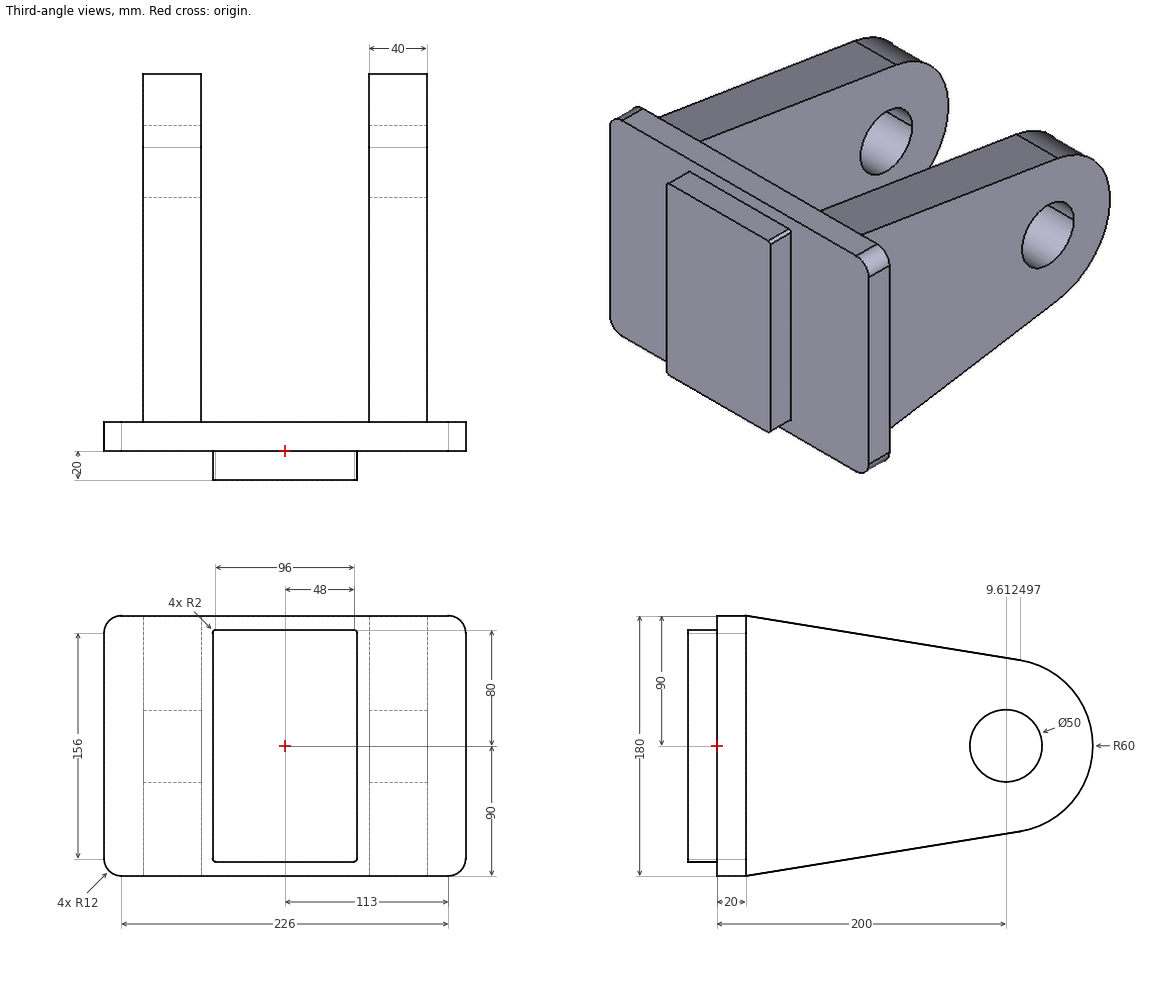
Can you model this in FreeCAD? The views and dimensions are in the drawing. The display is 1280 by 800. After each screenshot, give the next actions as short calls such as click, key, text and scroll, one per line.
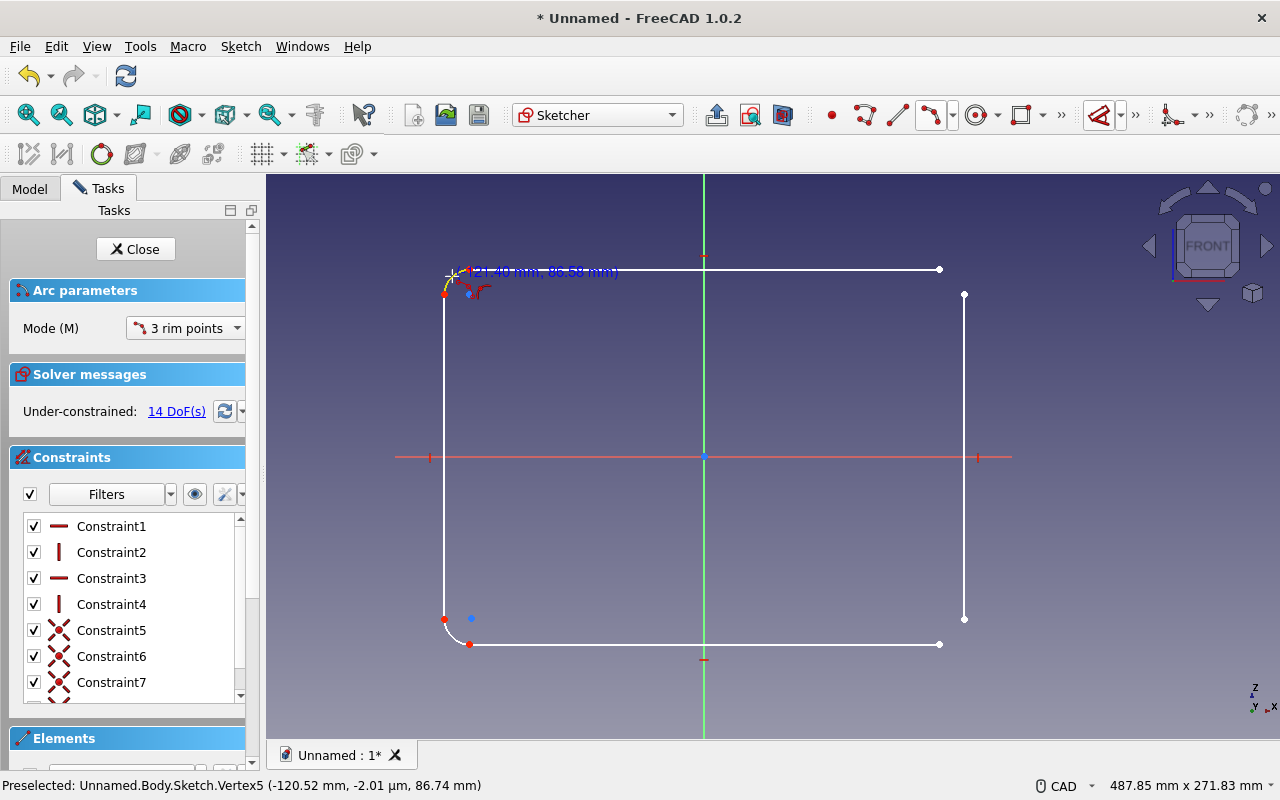
click(939, 270)
click(964, 295)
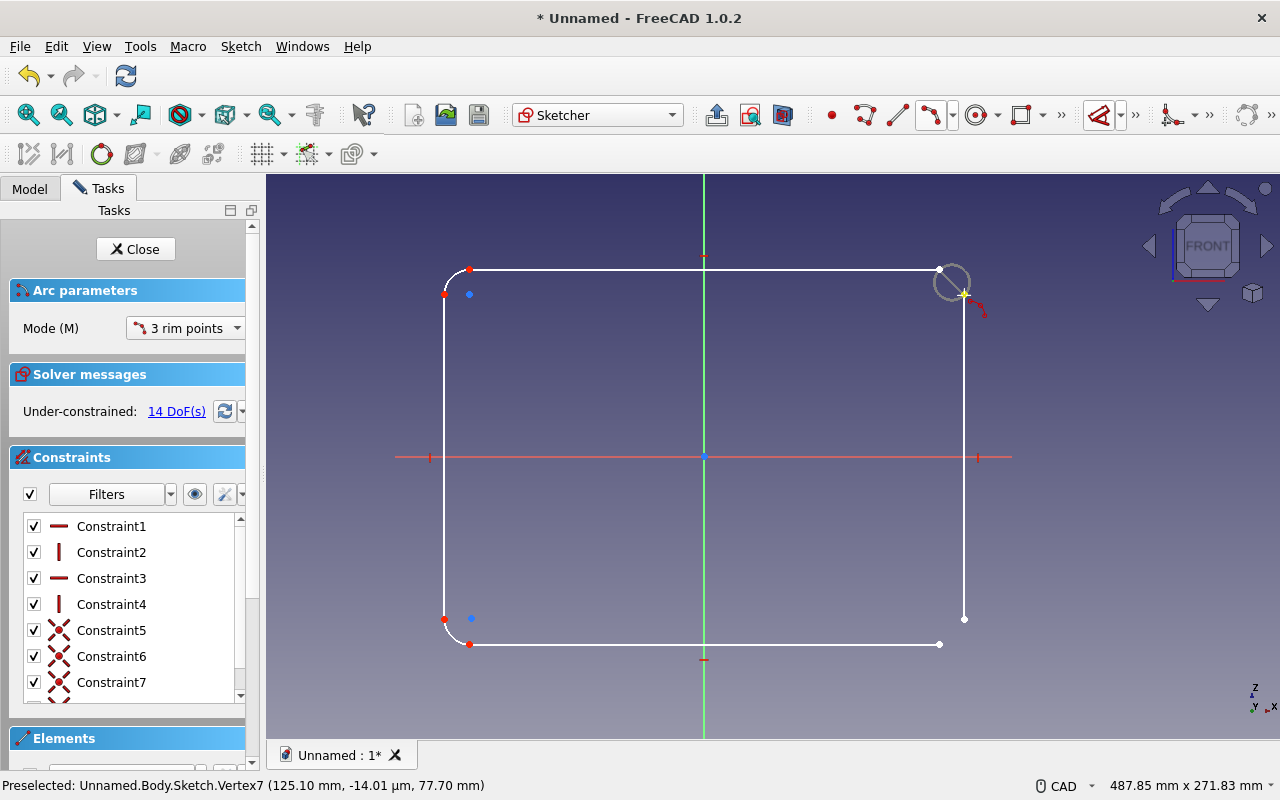
scroll(957, 277, up, 4)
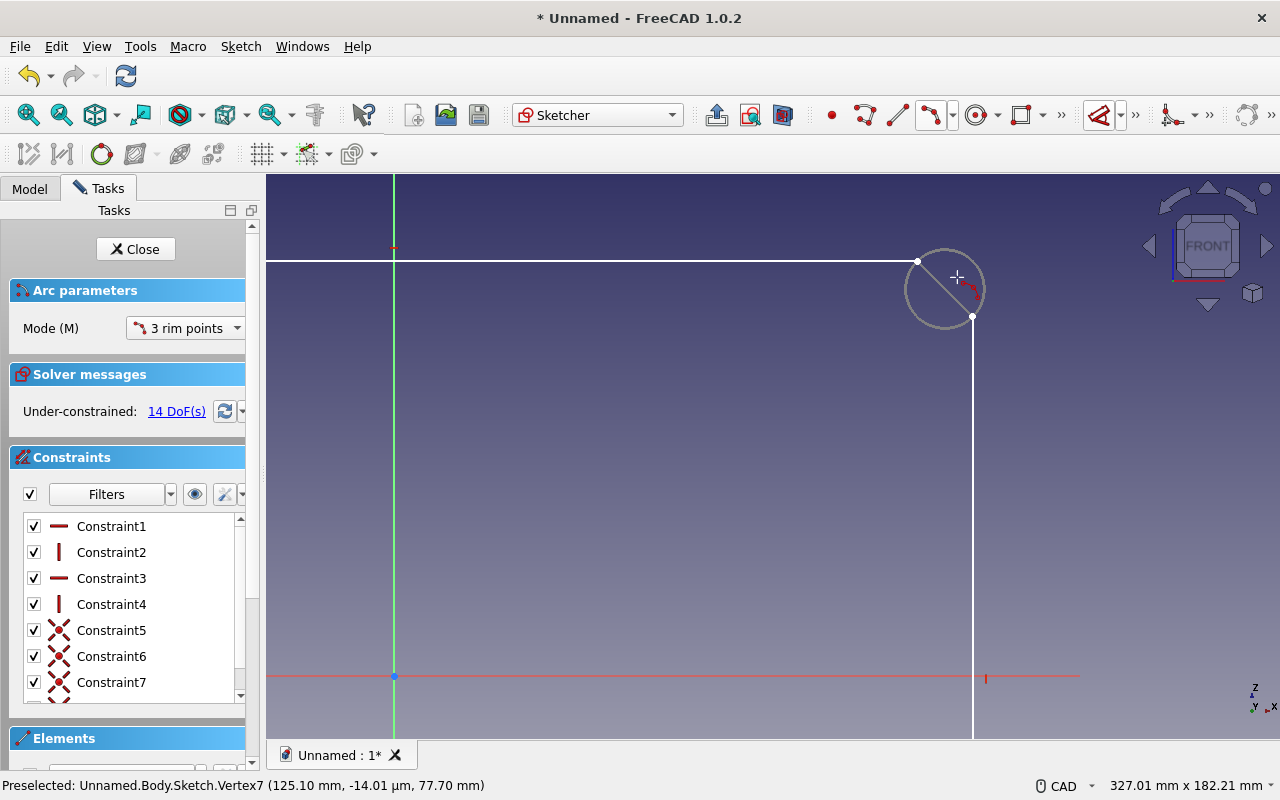
click(956, 276)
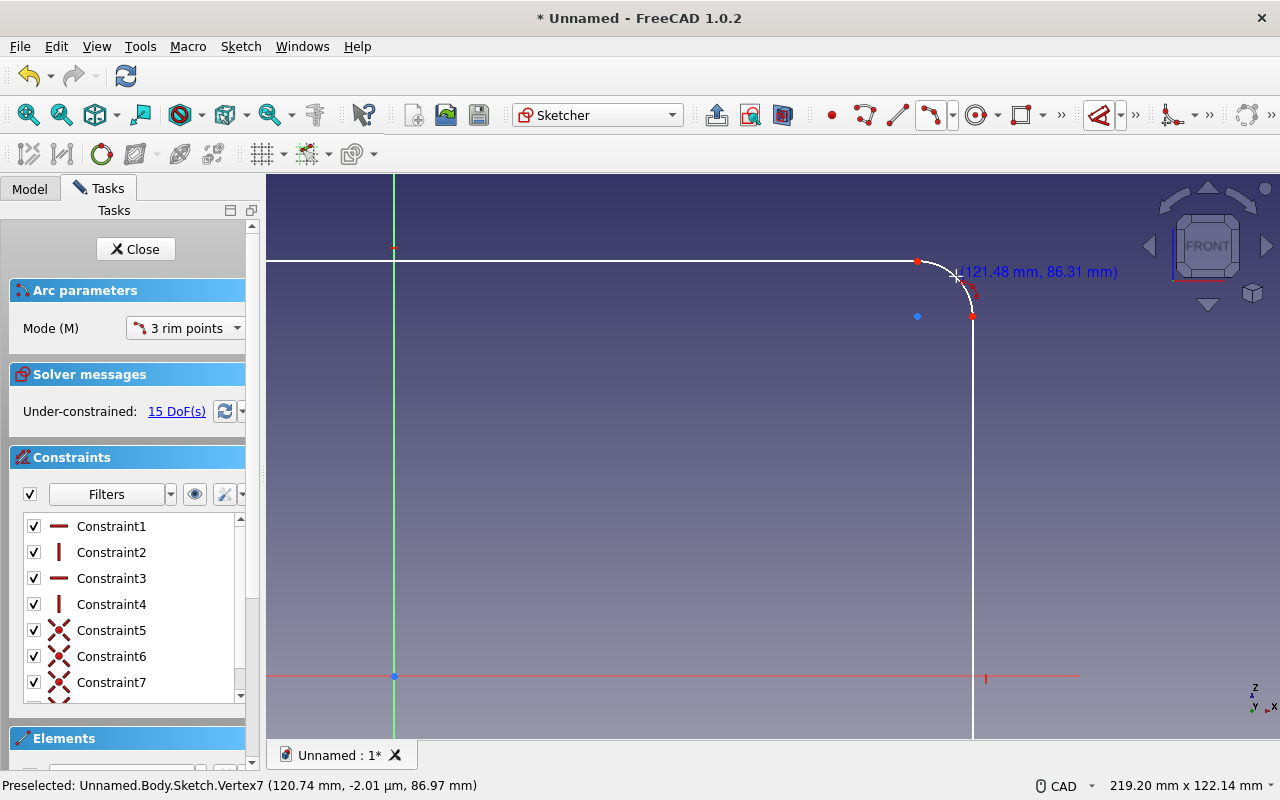
scroll(958, 277, down, 4)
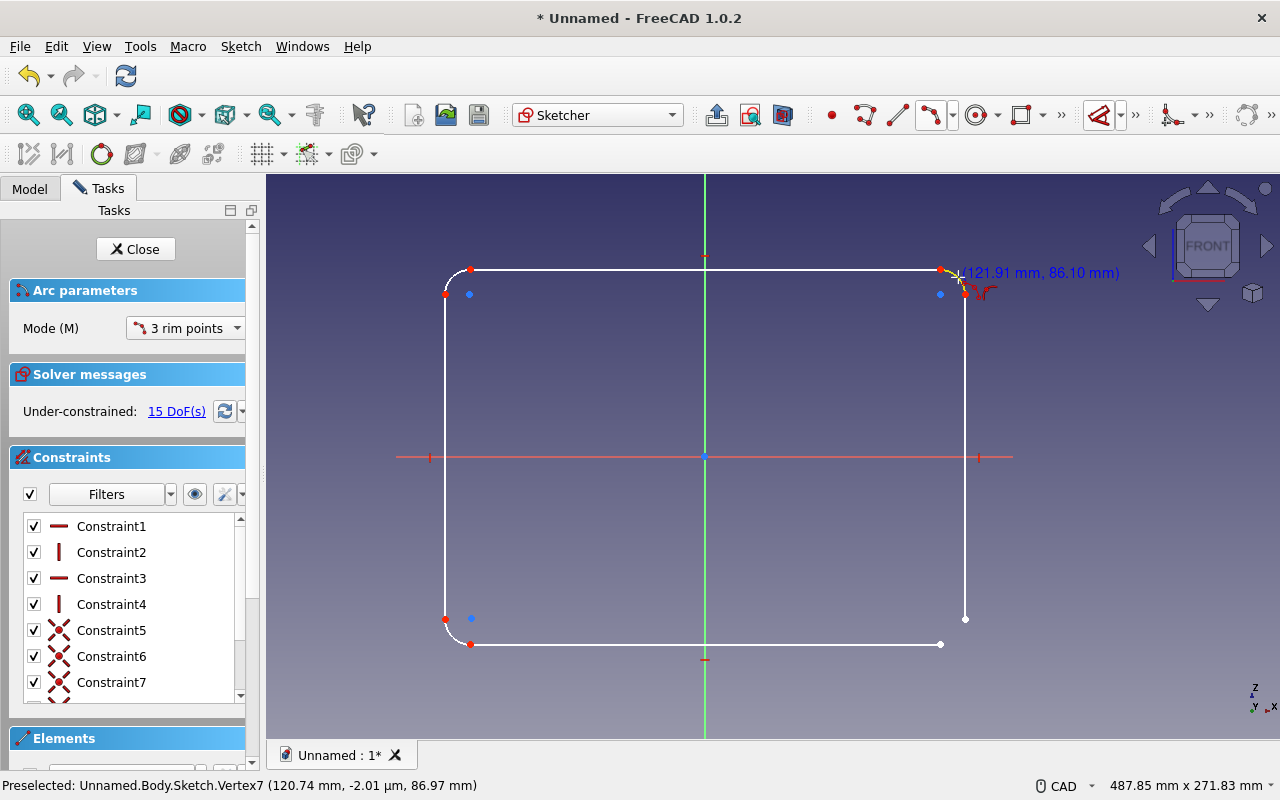
click(965, 620)
click(940, 645)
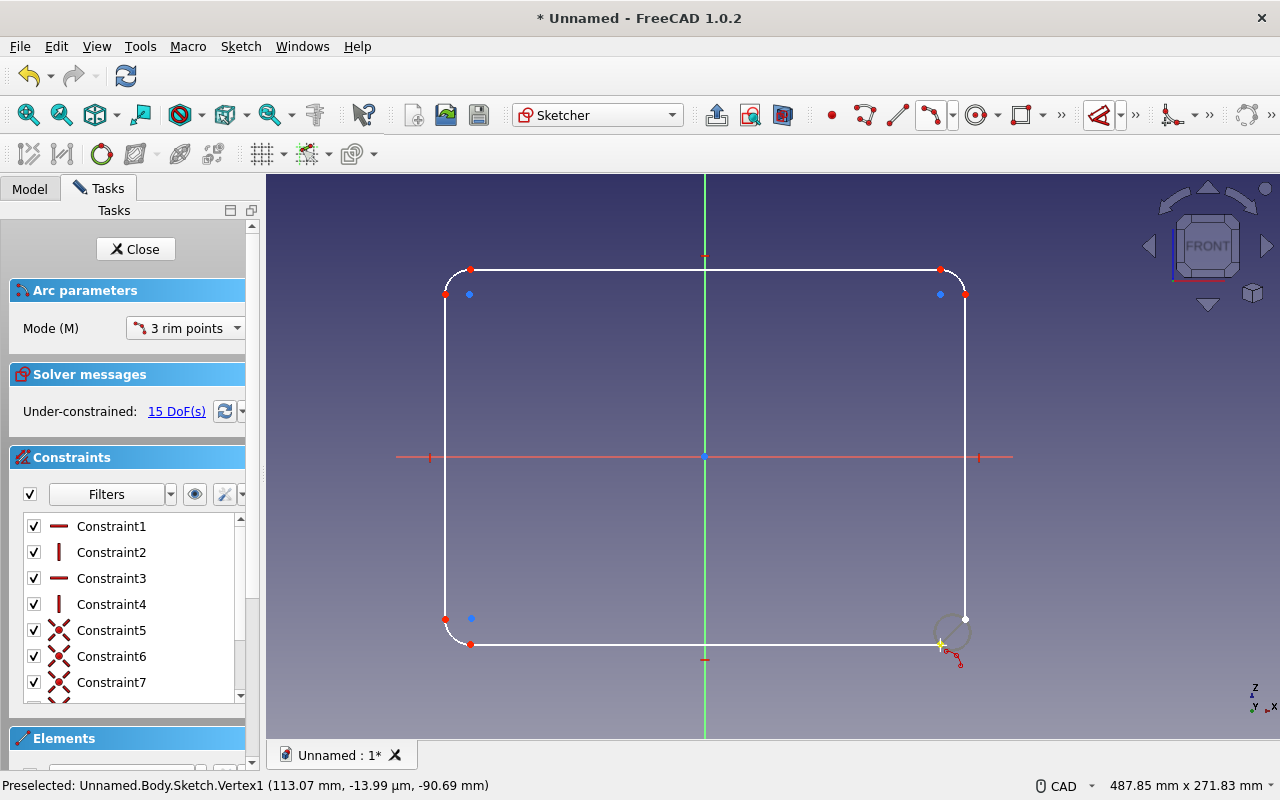
scroll(957, 636, up, 4)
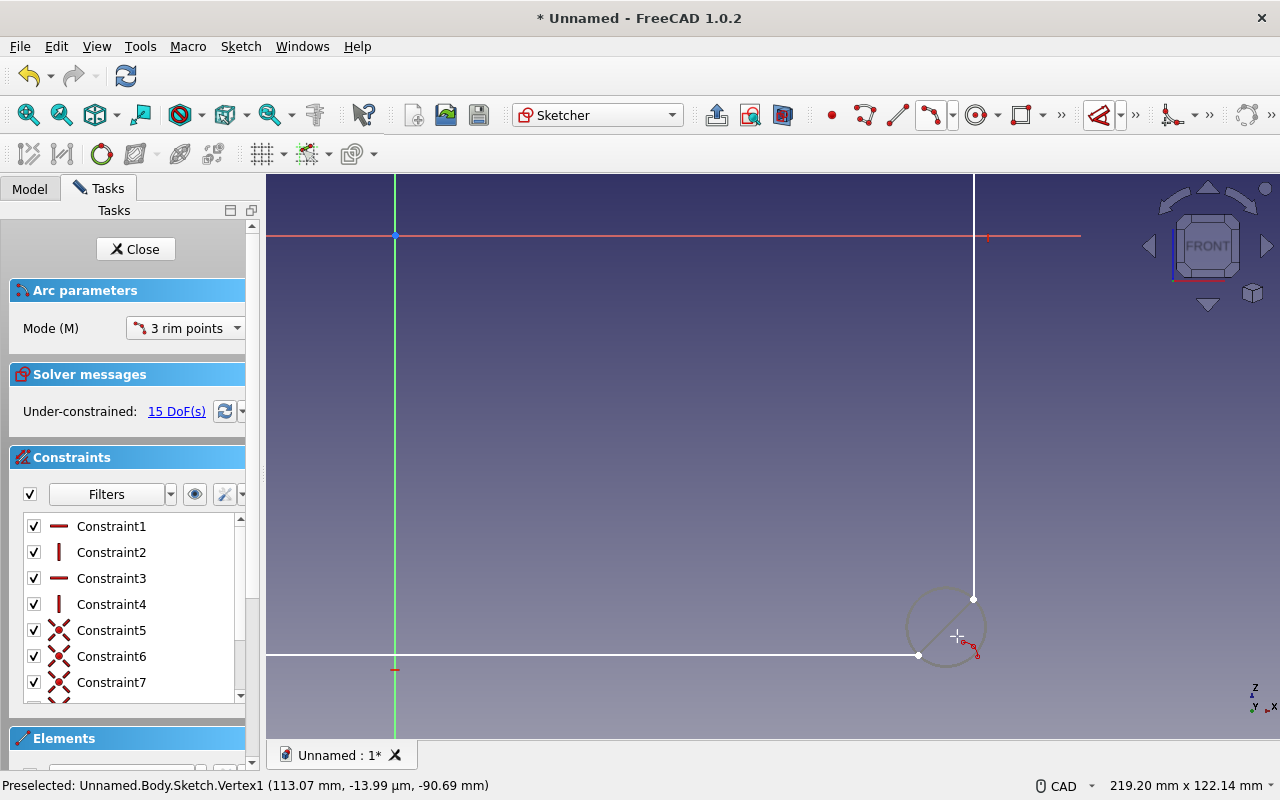
click(957, 636)
key(Escape)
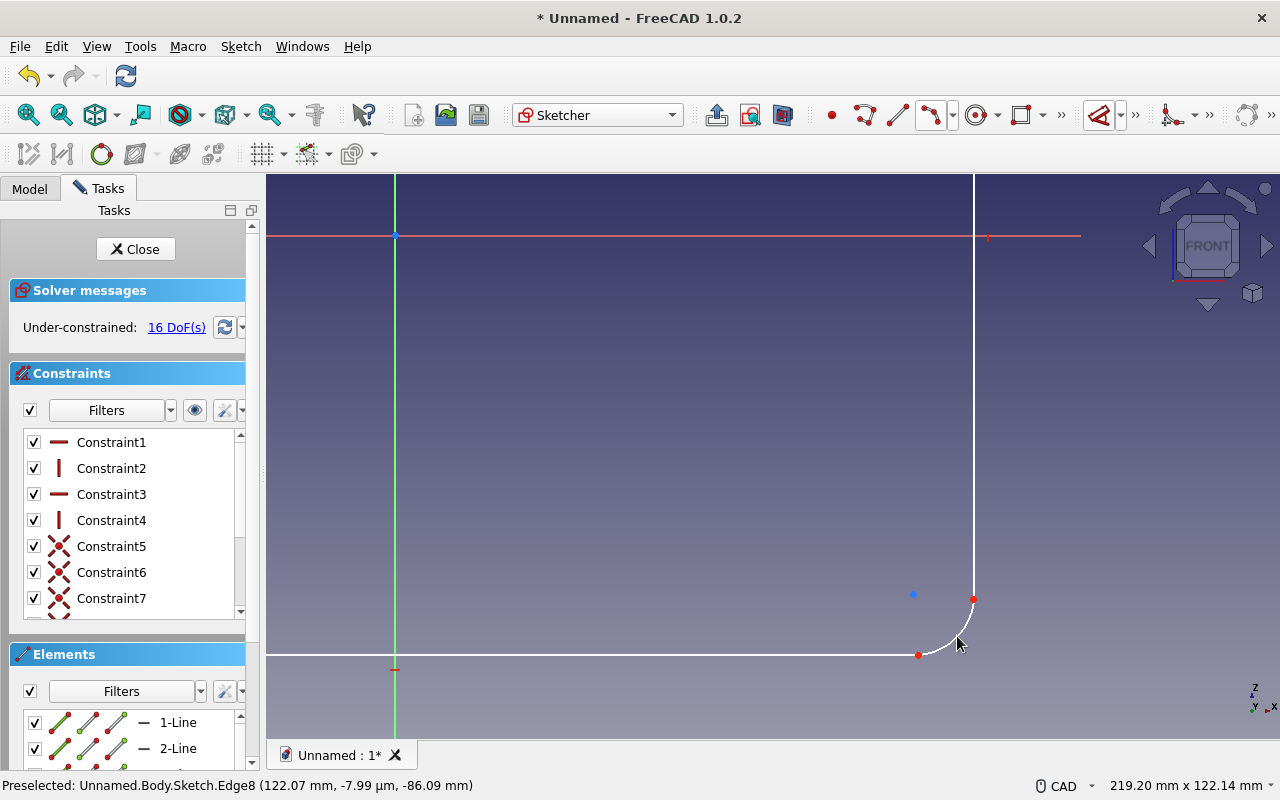
click(605, 655)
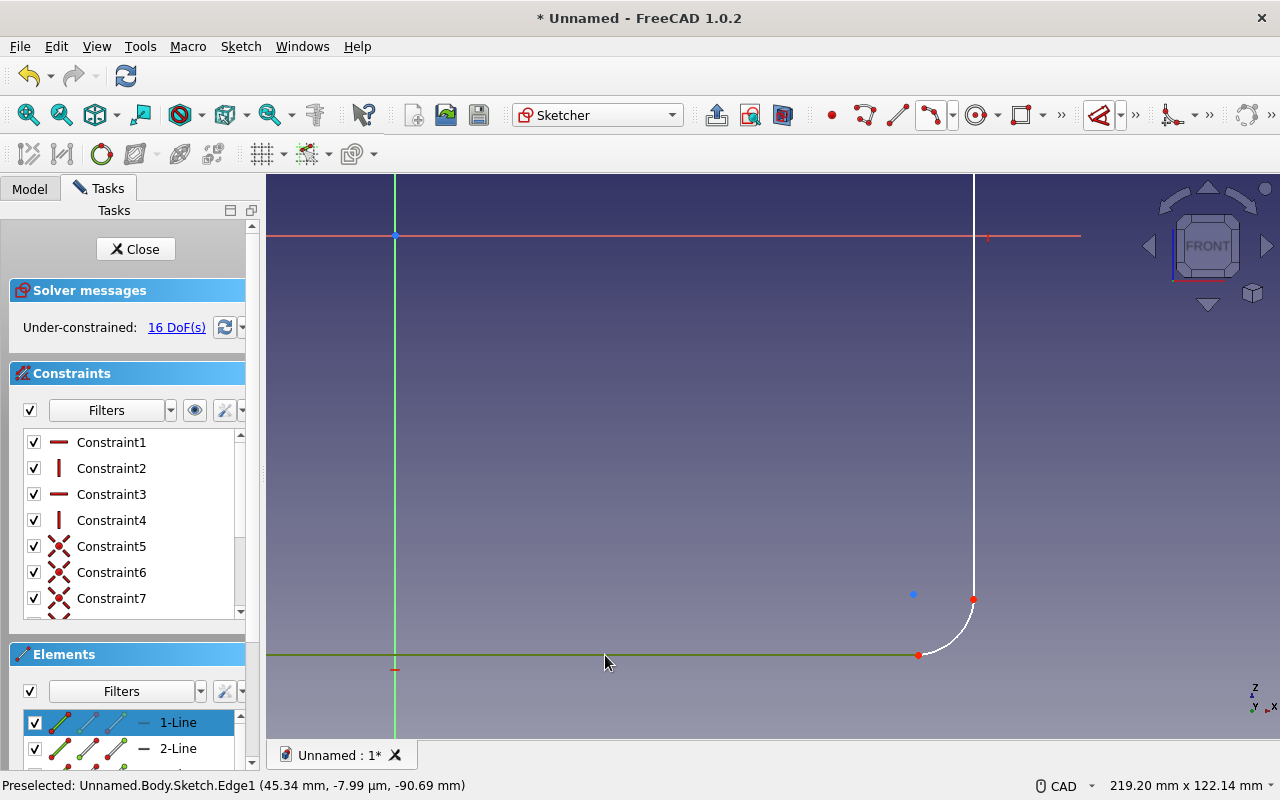
scroll(957, 637, down, 4)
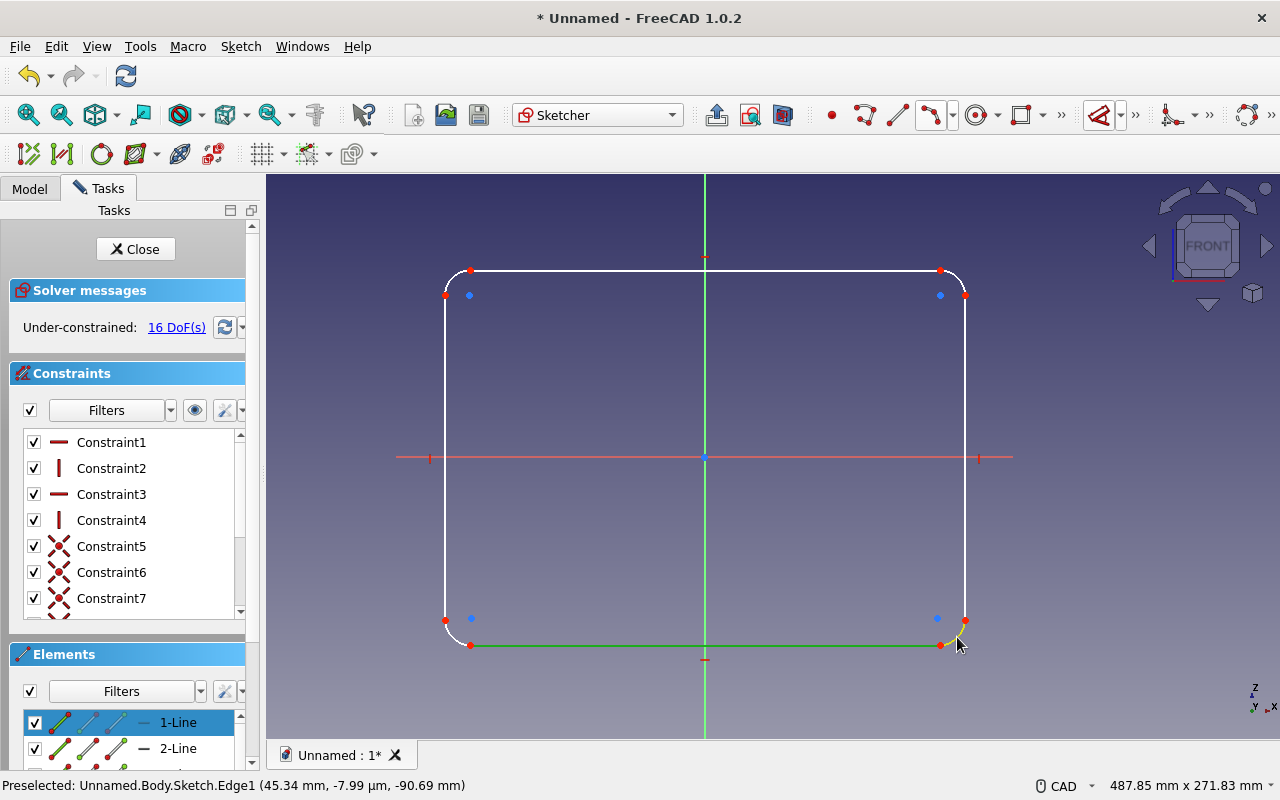
click(448, 632)